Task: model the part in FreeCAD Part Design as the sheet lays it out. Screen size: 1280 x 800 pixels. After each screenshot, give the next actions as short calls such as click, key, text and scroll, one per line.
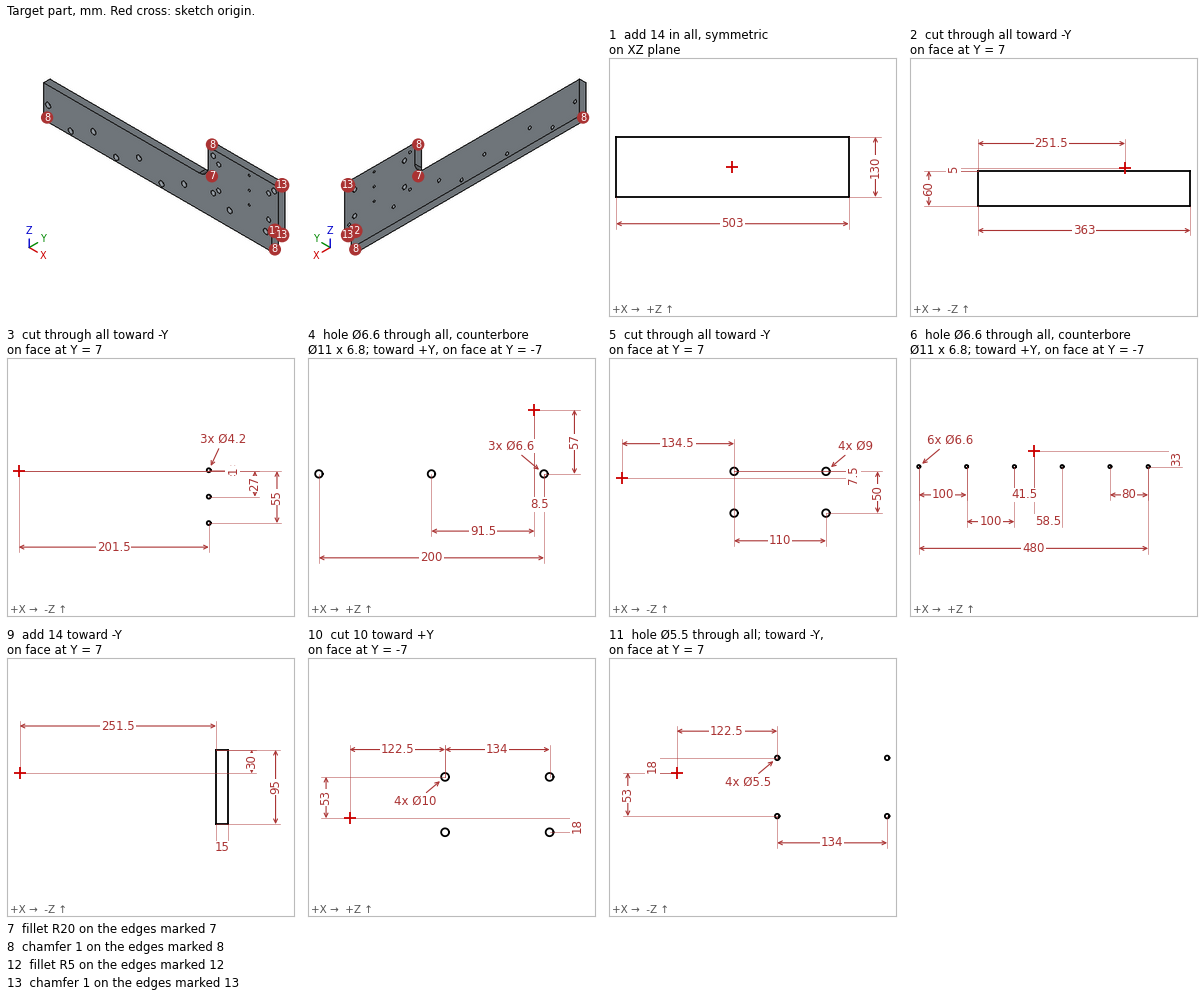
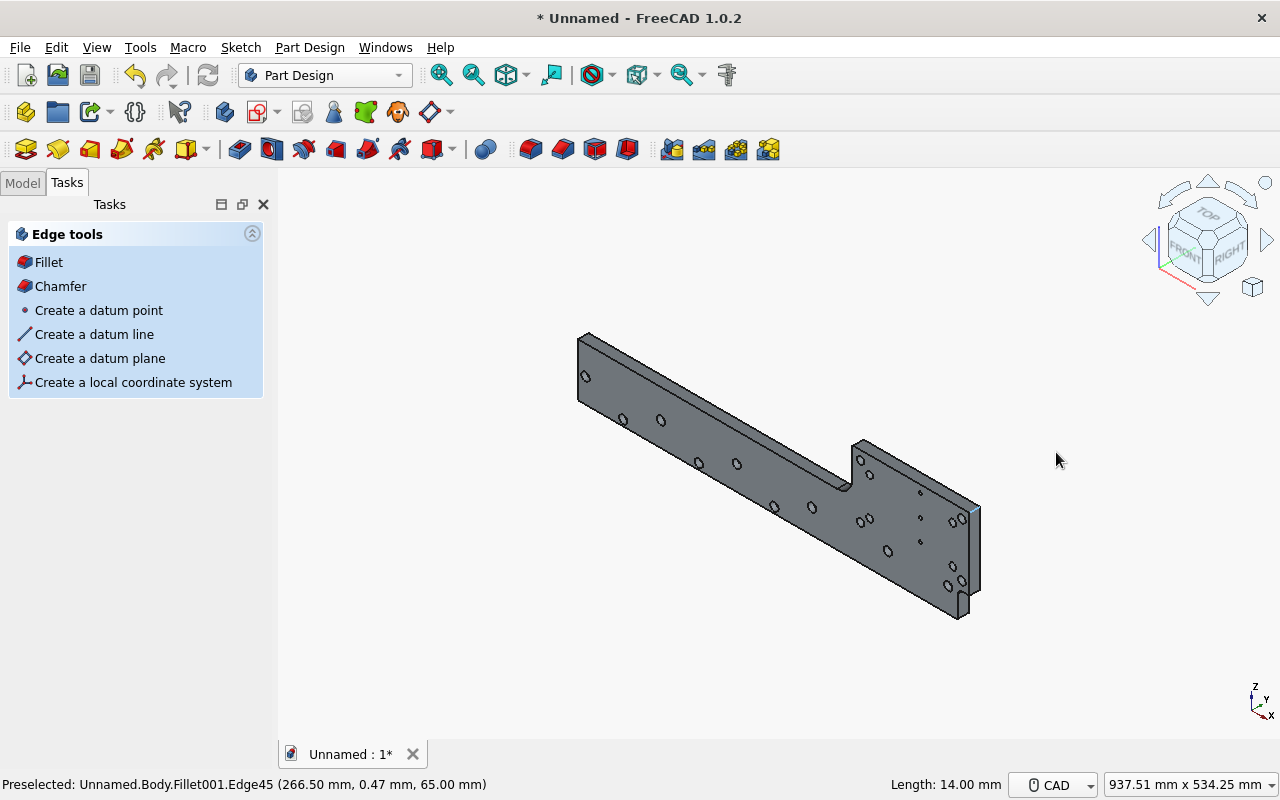
scroll(975, 592, up, 5)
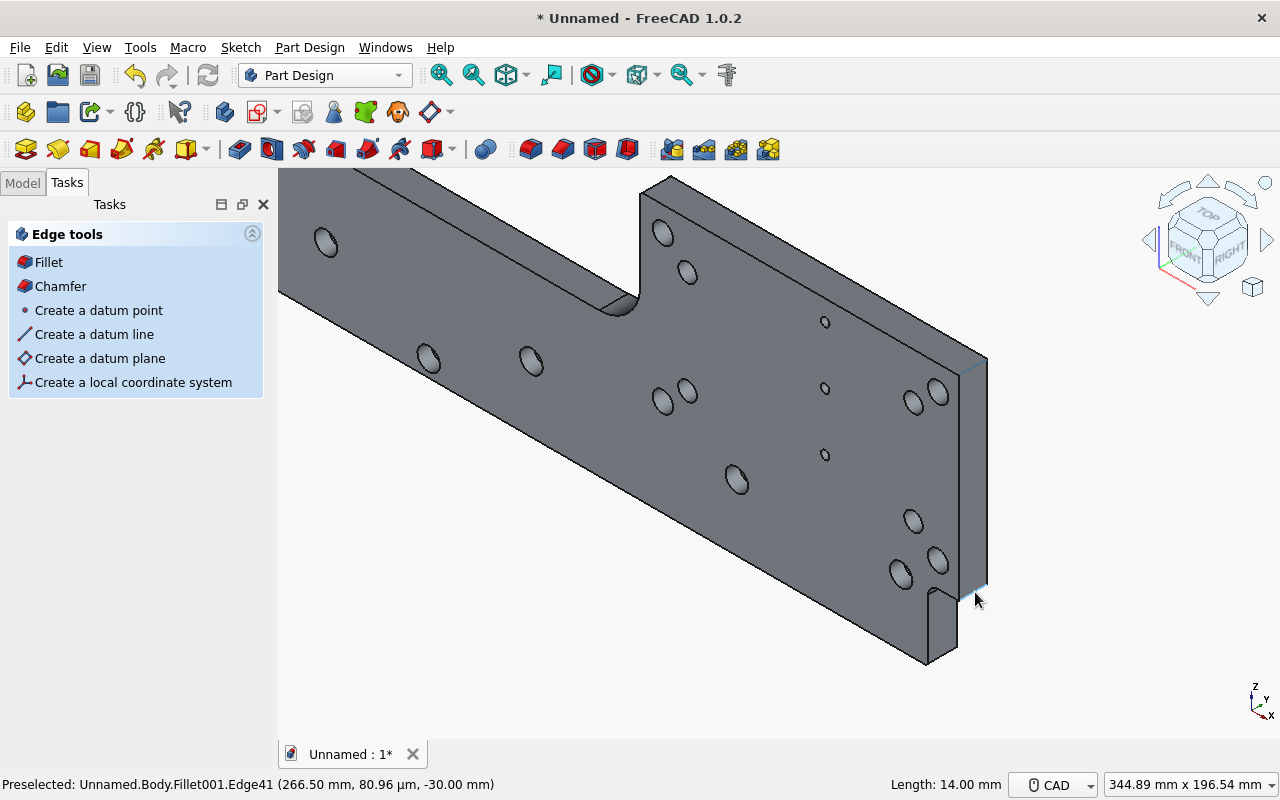
key(v)
key(f)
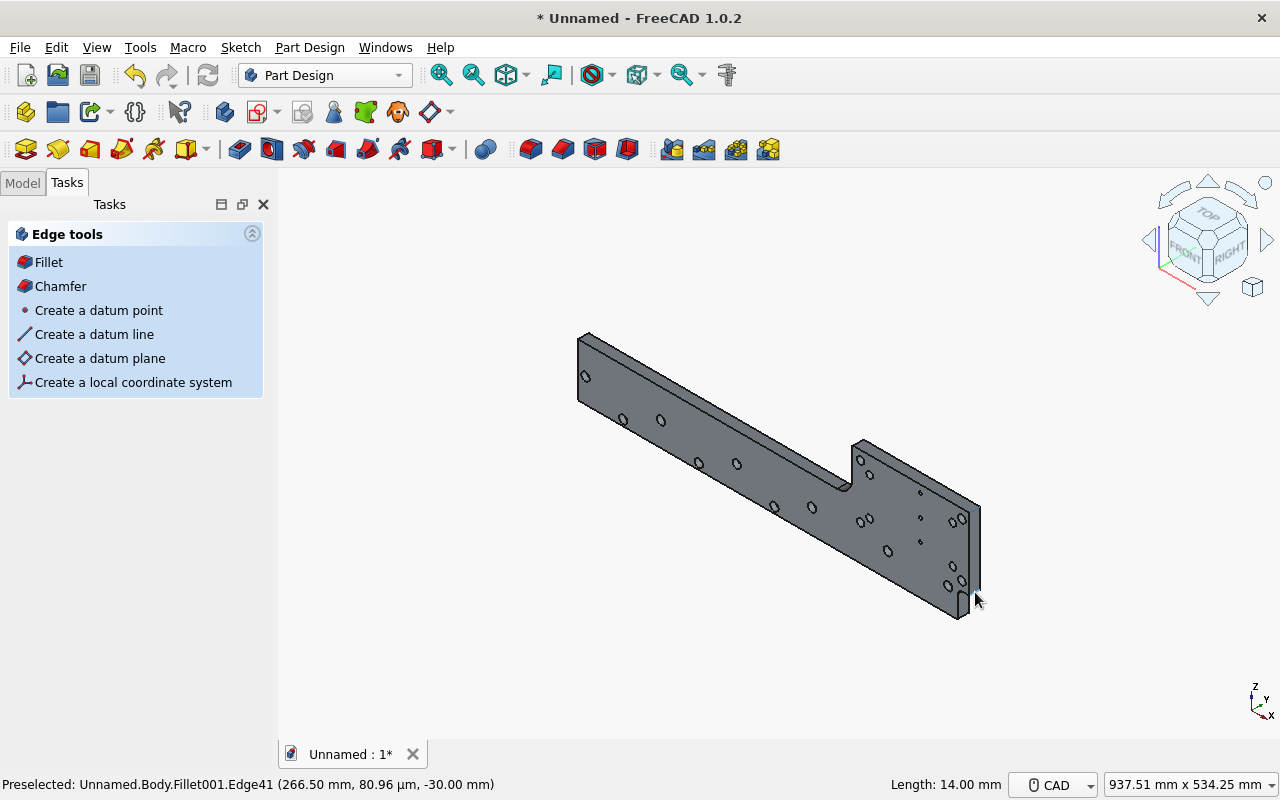
key(1)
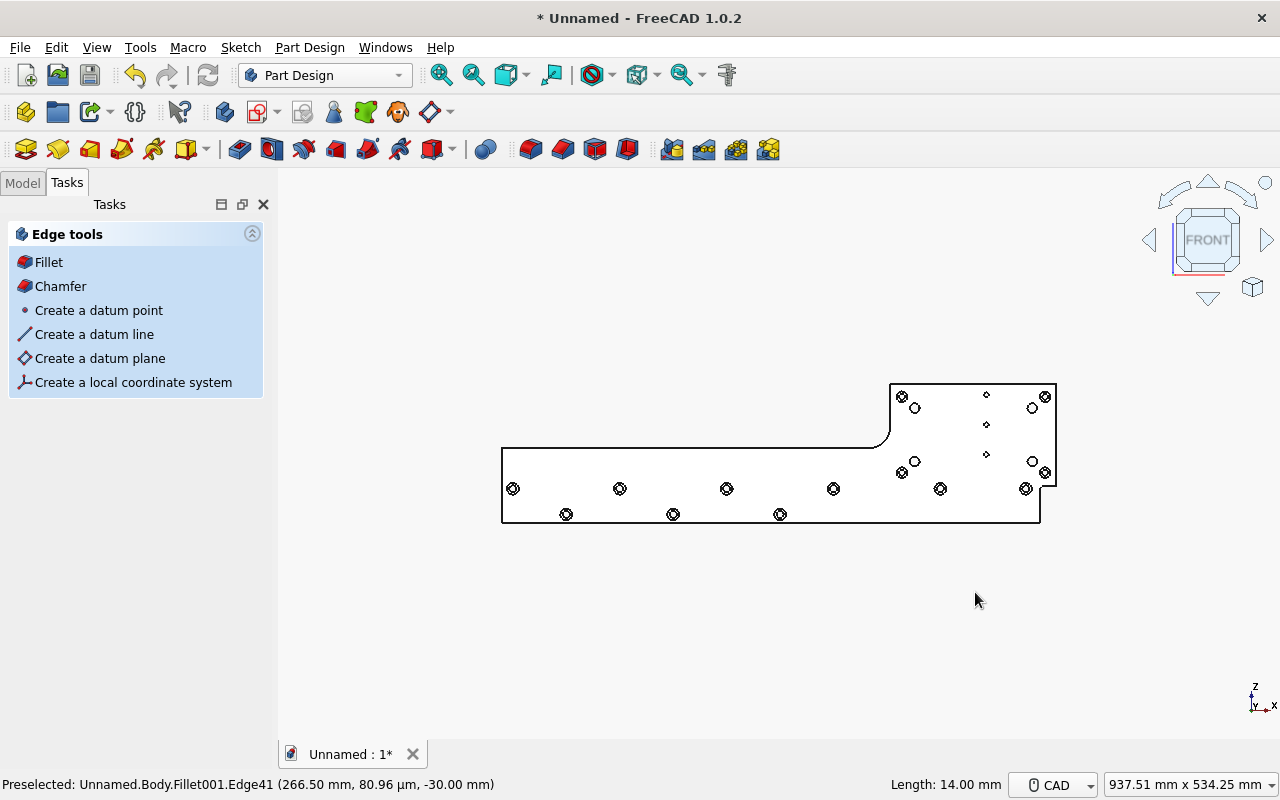
scroll(1056, 485, up, 5)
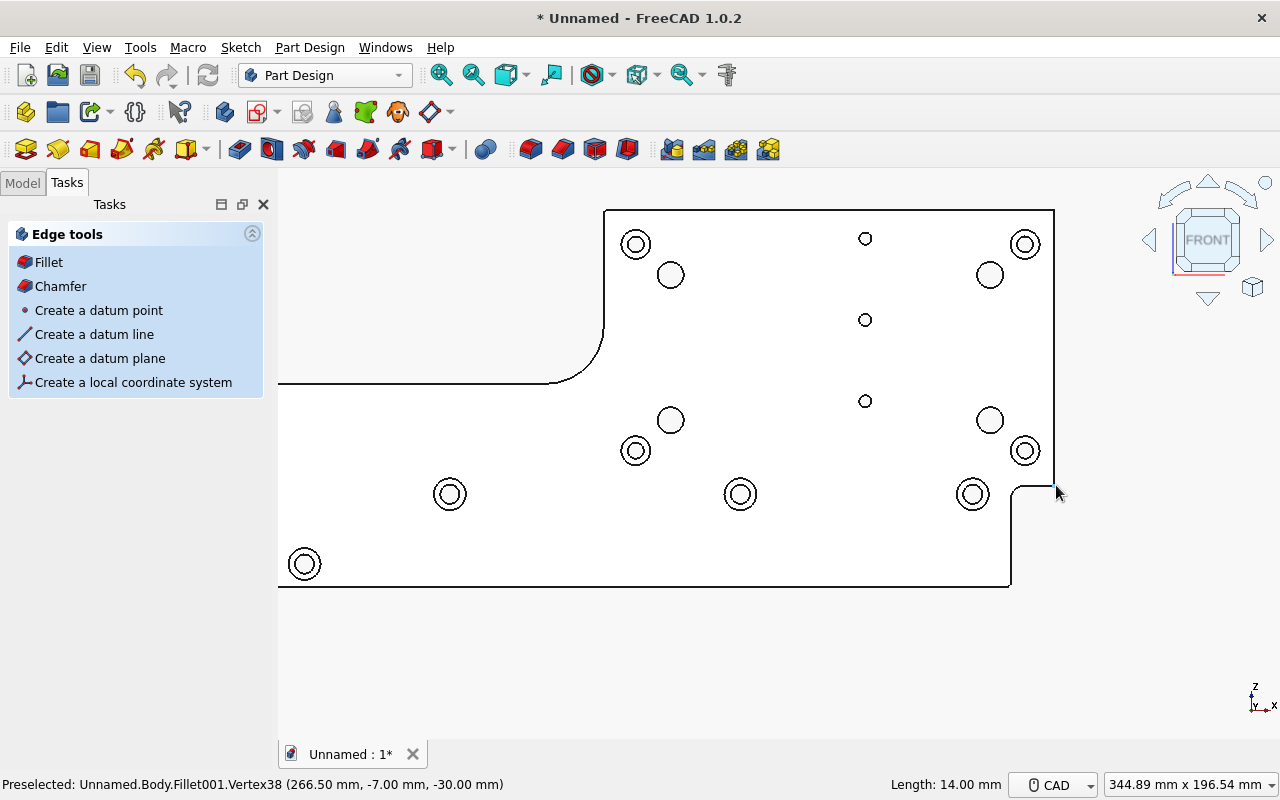
key(v)
key(f)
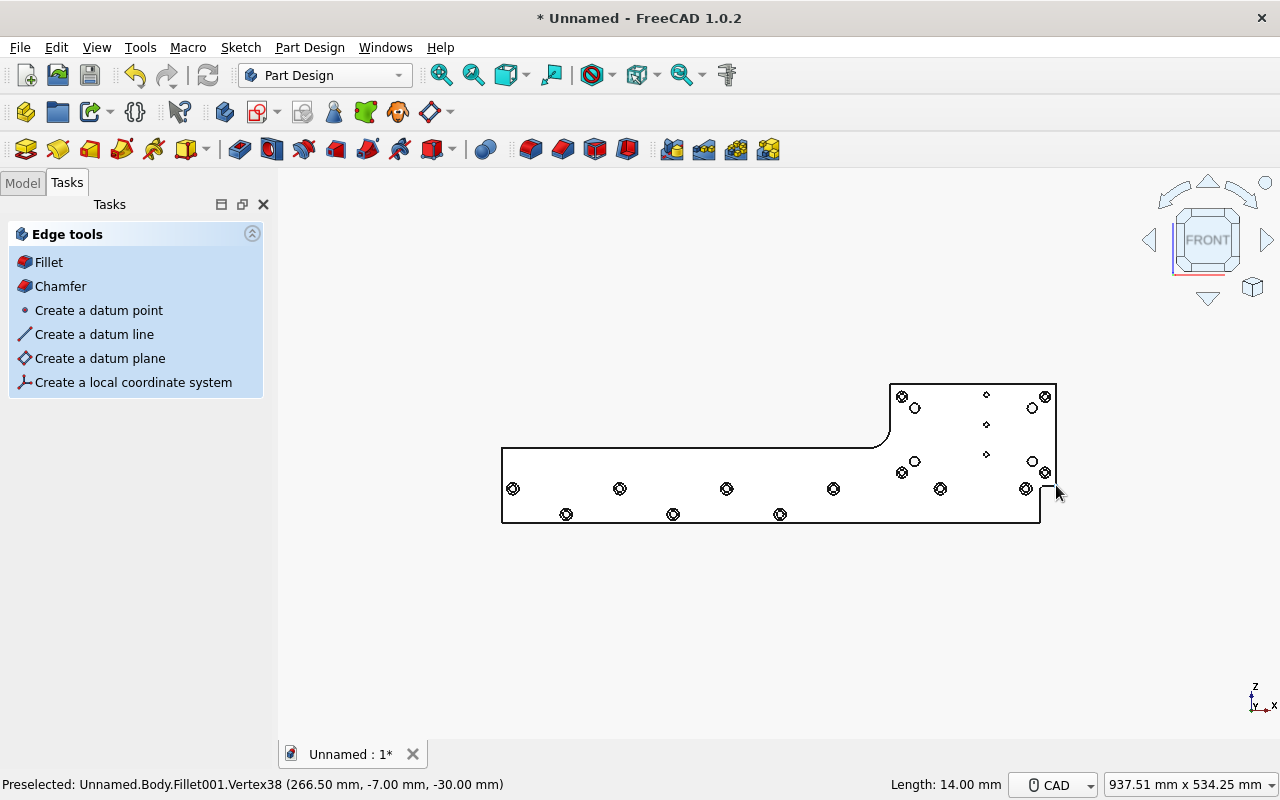
key(3)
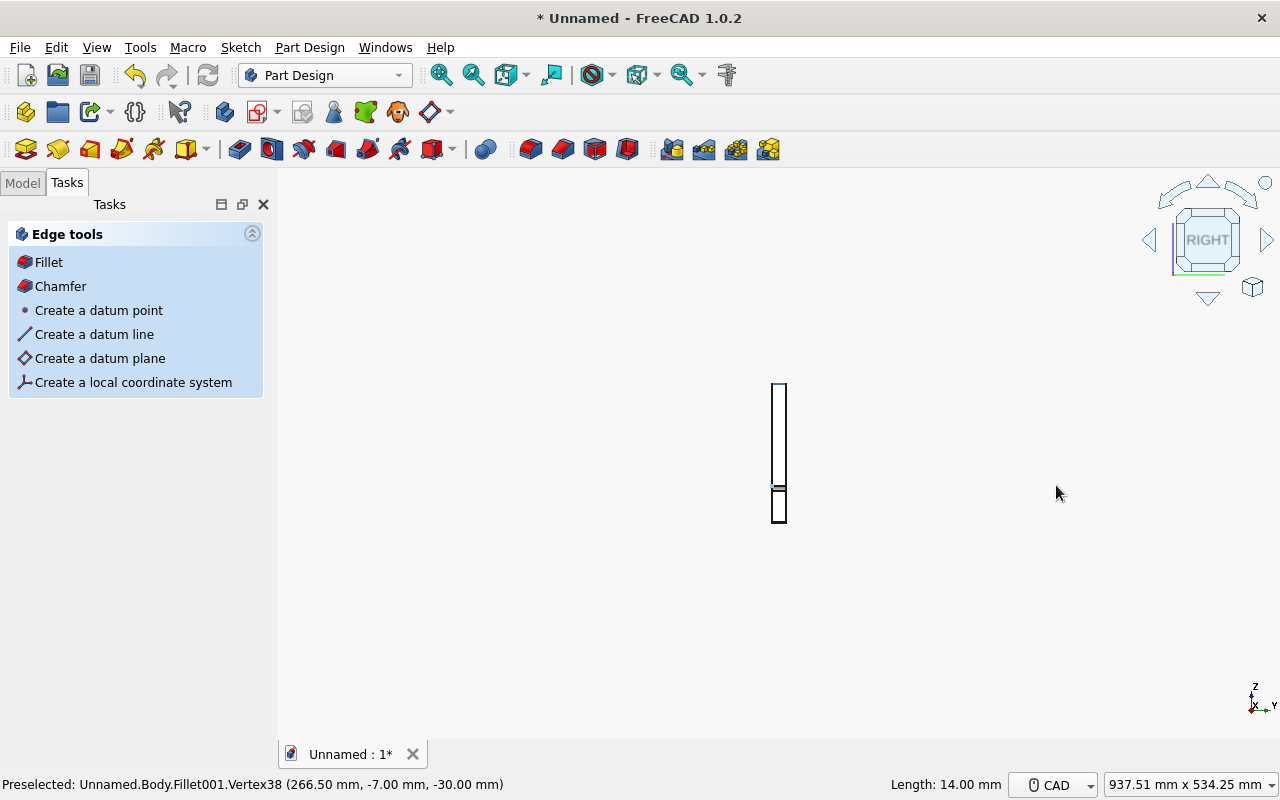
key(v)
key(f)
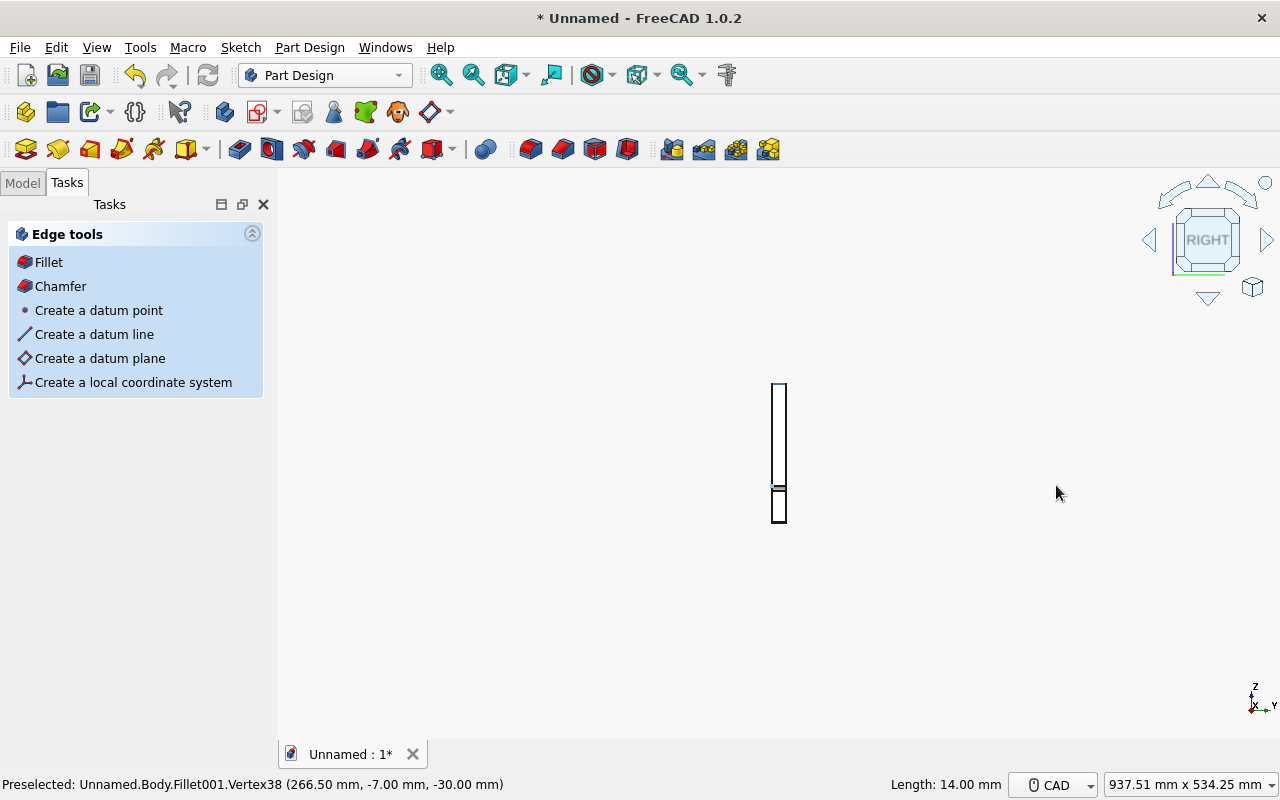
click(779, 485, ctrl)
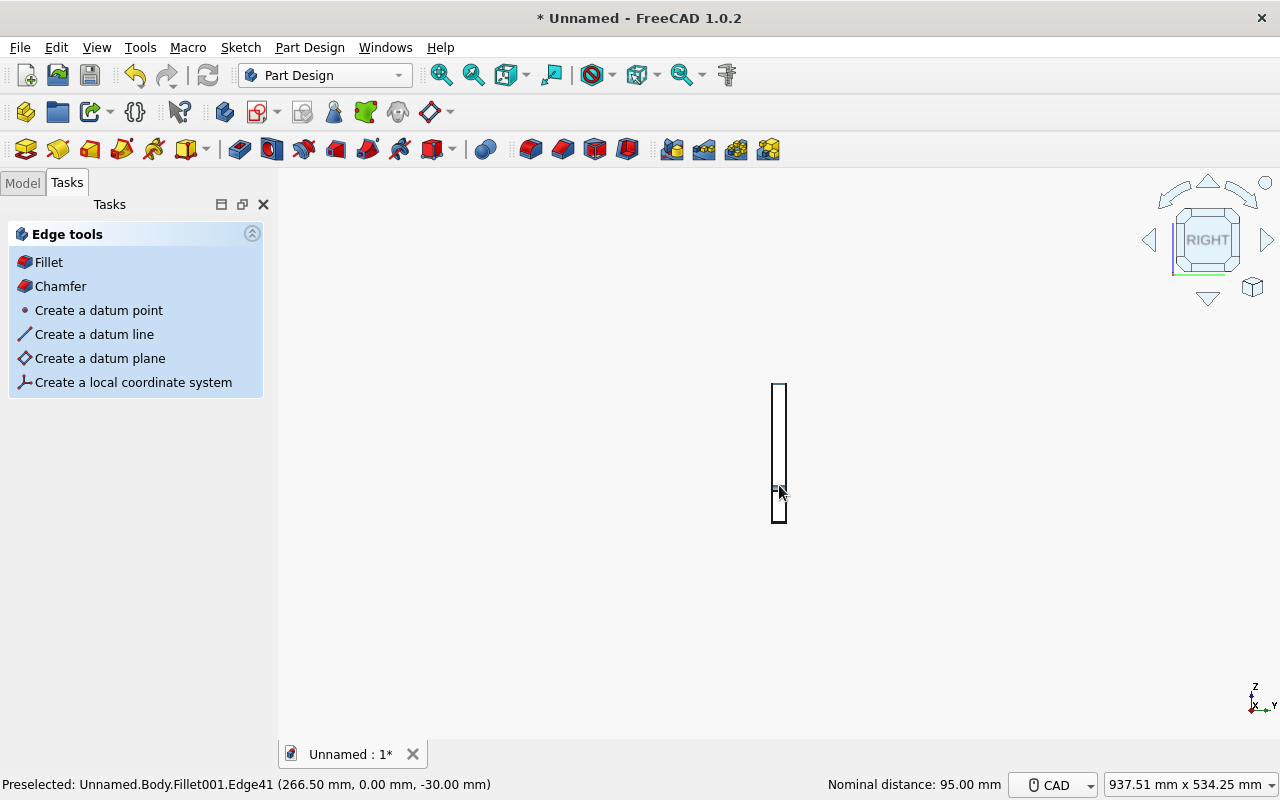
click(564, 150)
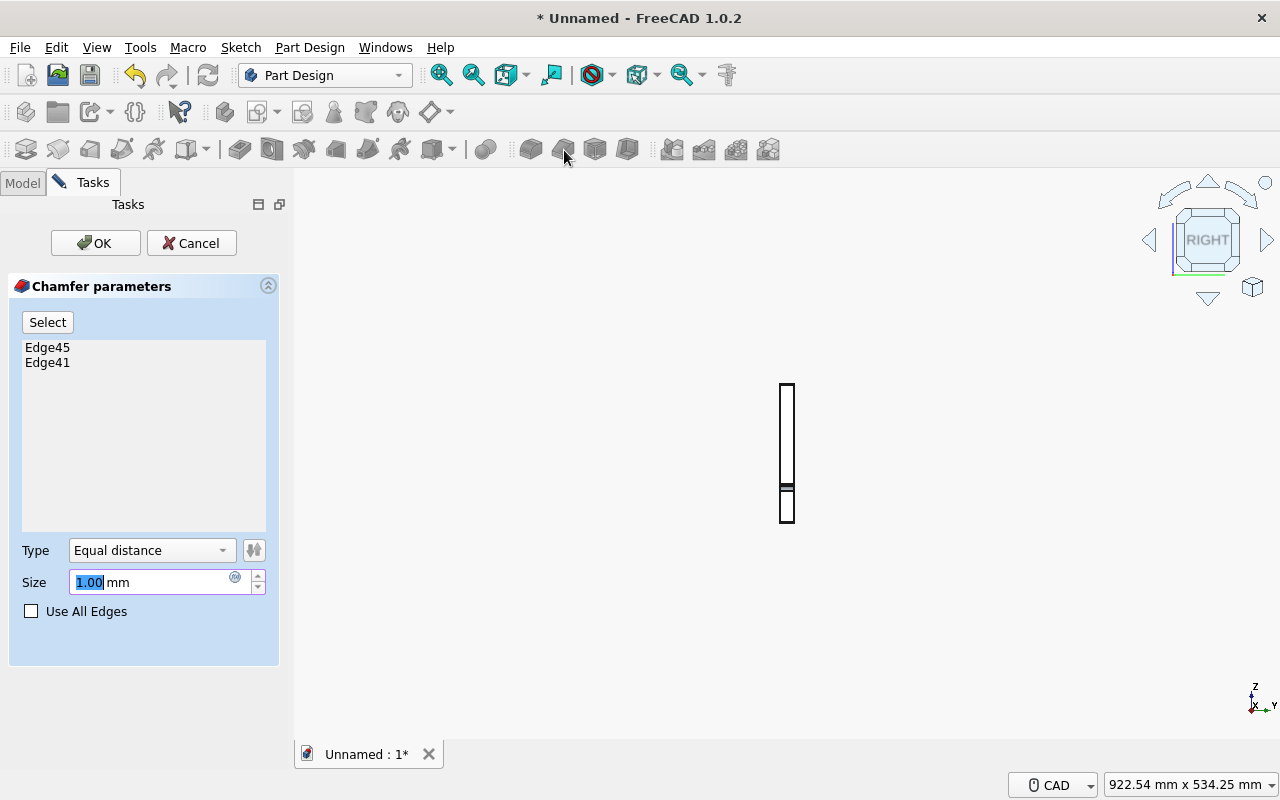
text(1)
key(Tab)